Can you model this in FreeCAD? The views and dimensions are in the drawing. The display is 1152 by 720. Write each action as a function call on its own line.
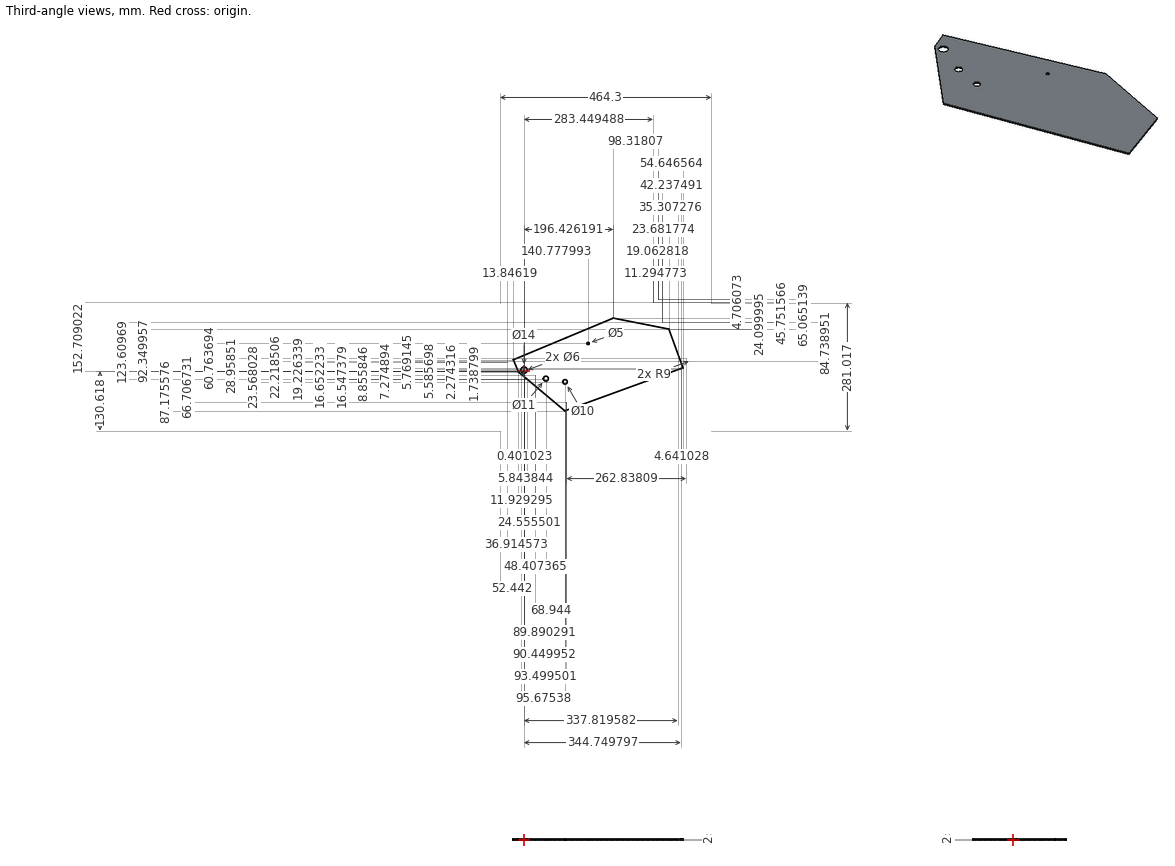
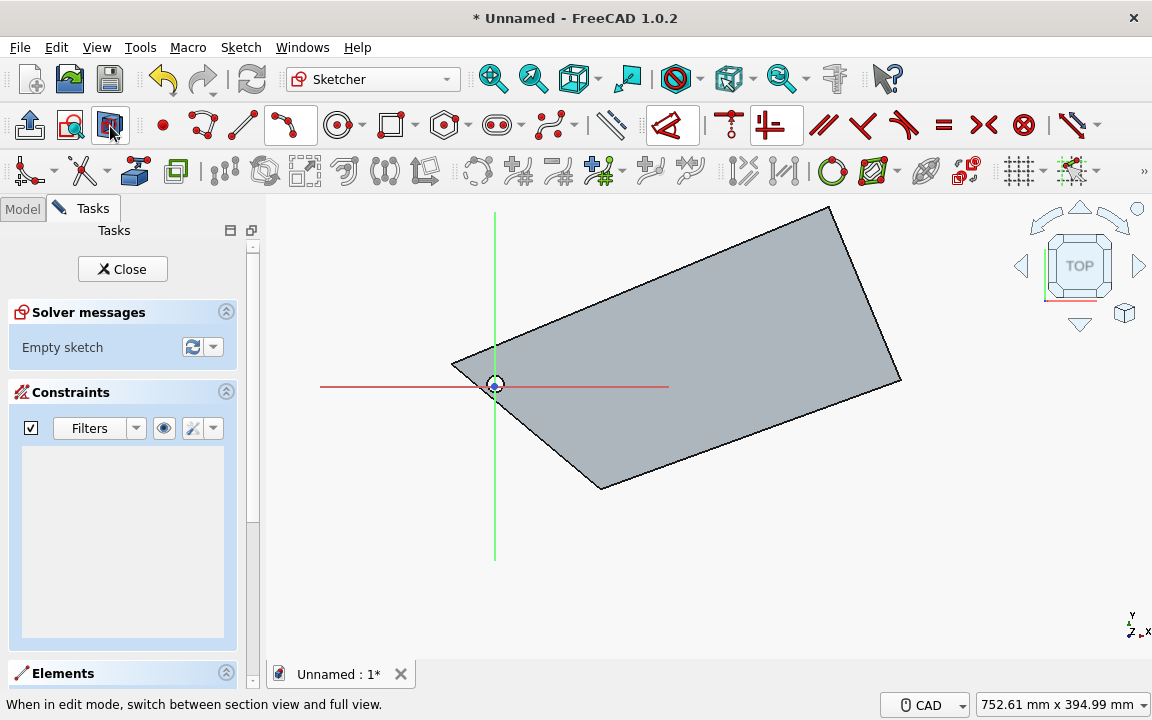
scroll(369, 631, down, 1)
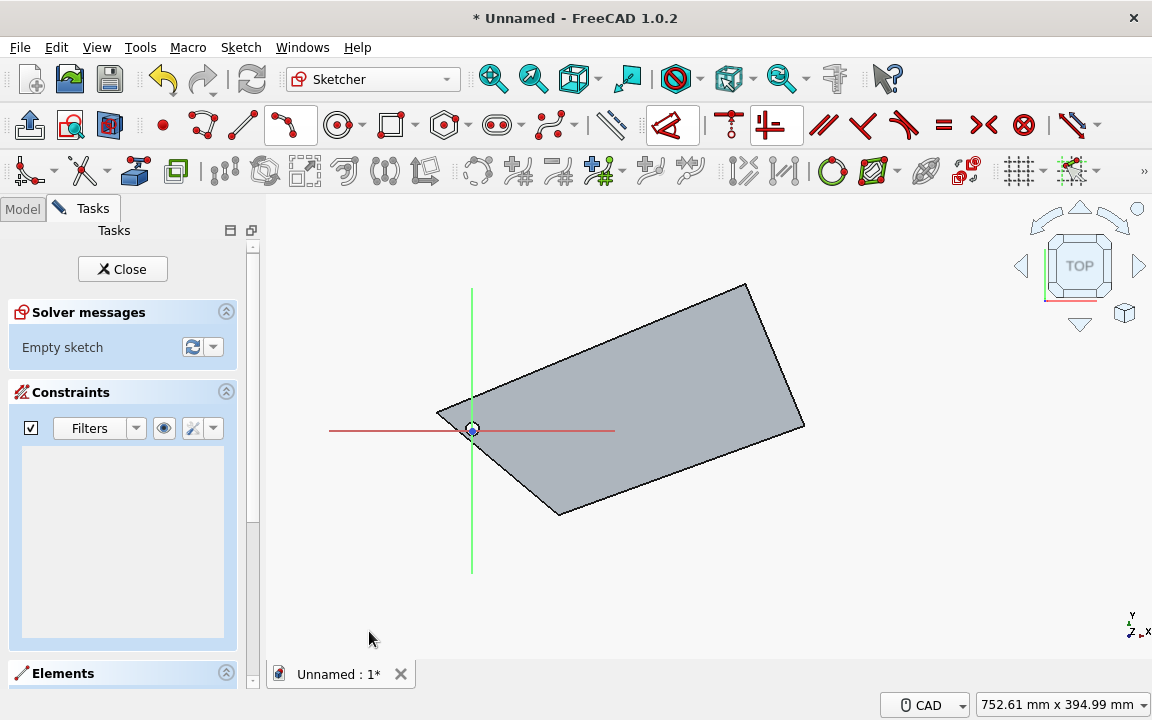
scroll(641, 222, up, 2)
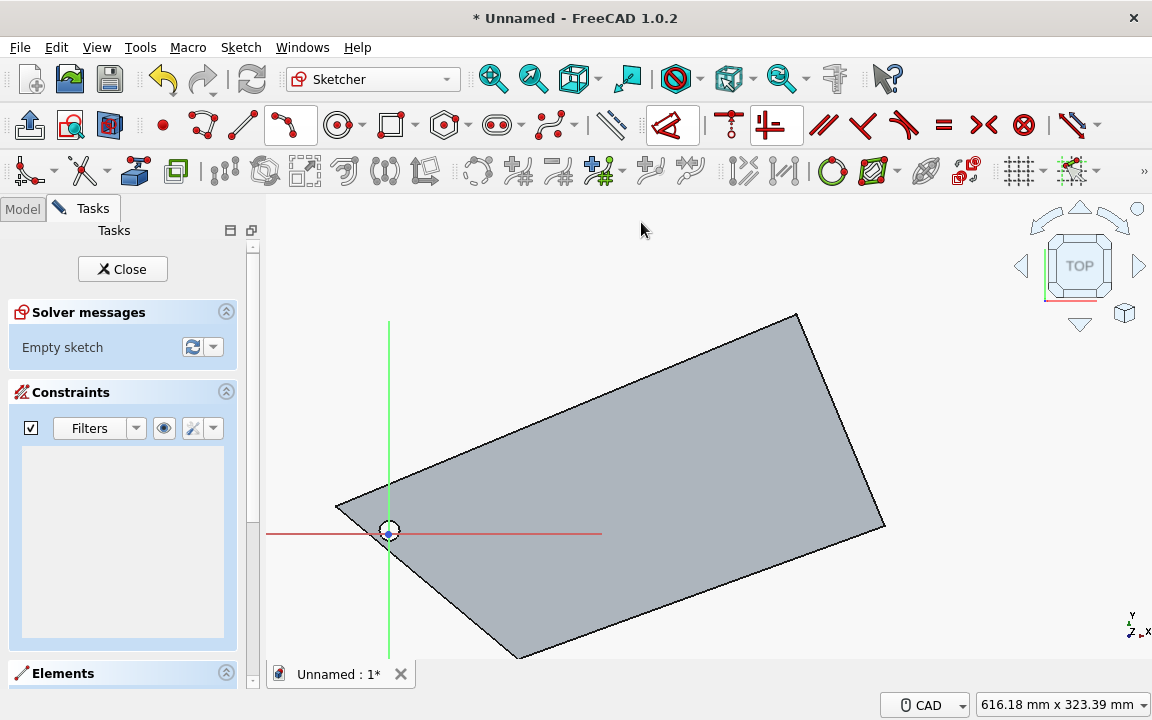
key(g)
key(m)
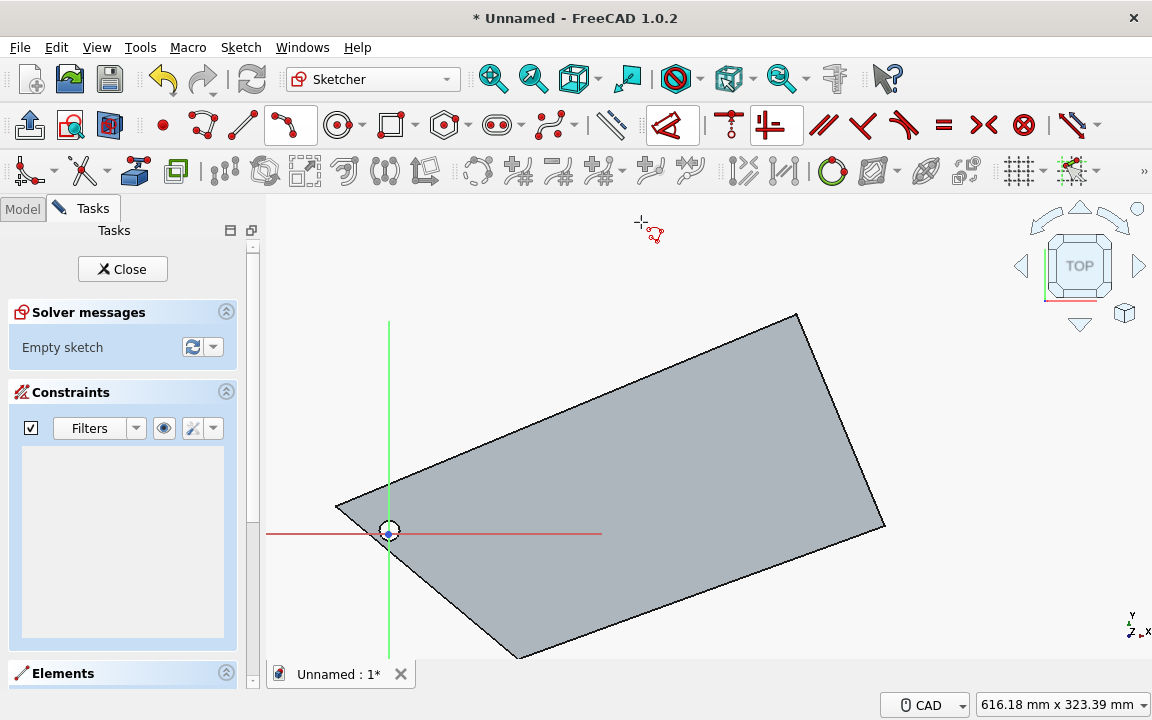
click(796, 314)
click(813, 308)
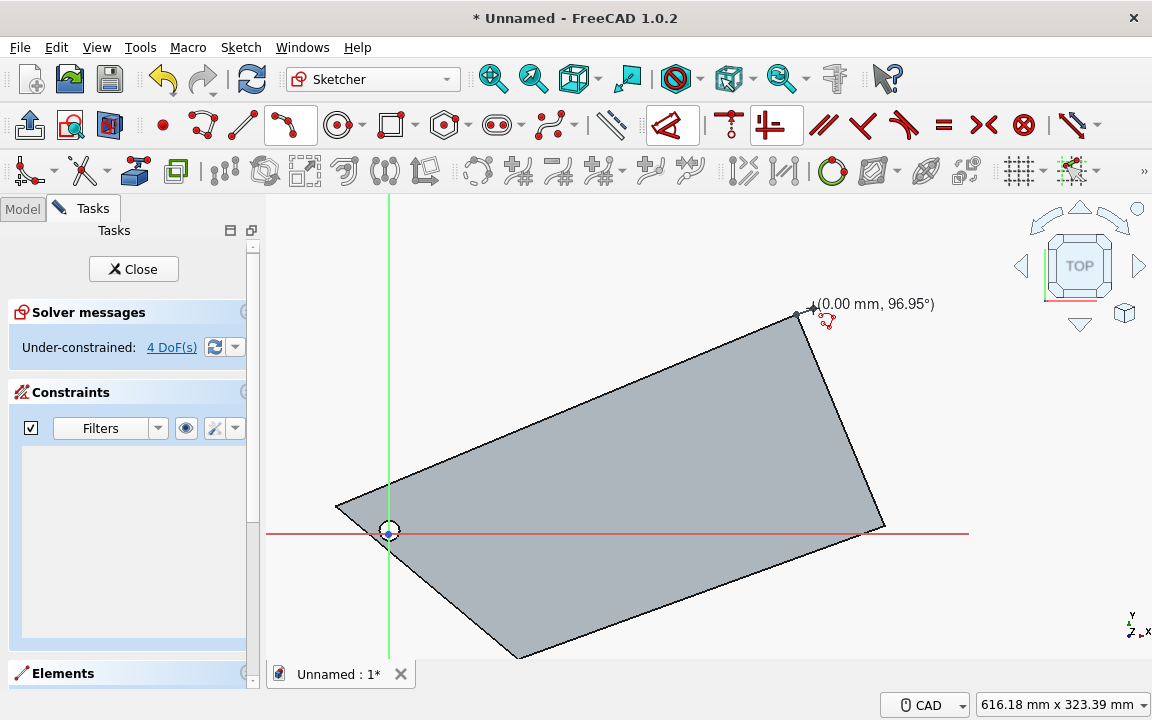
scroll(891, 524, up, 3)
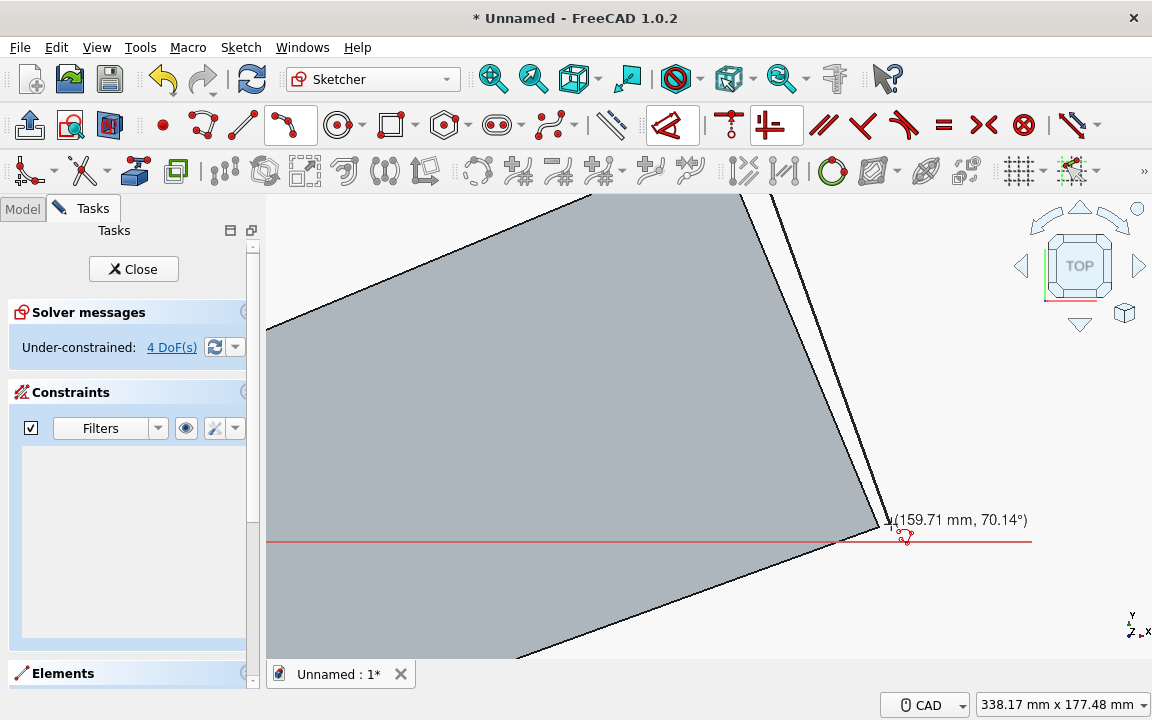
click(891, 523)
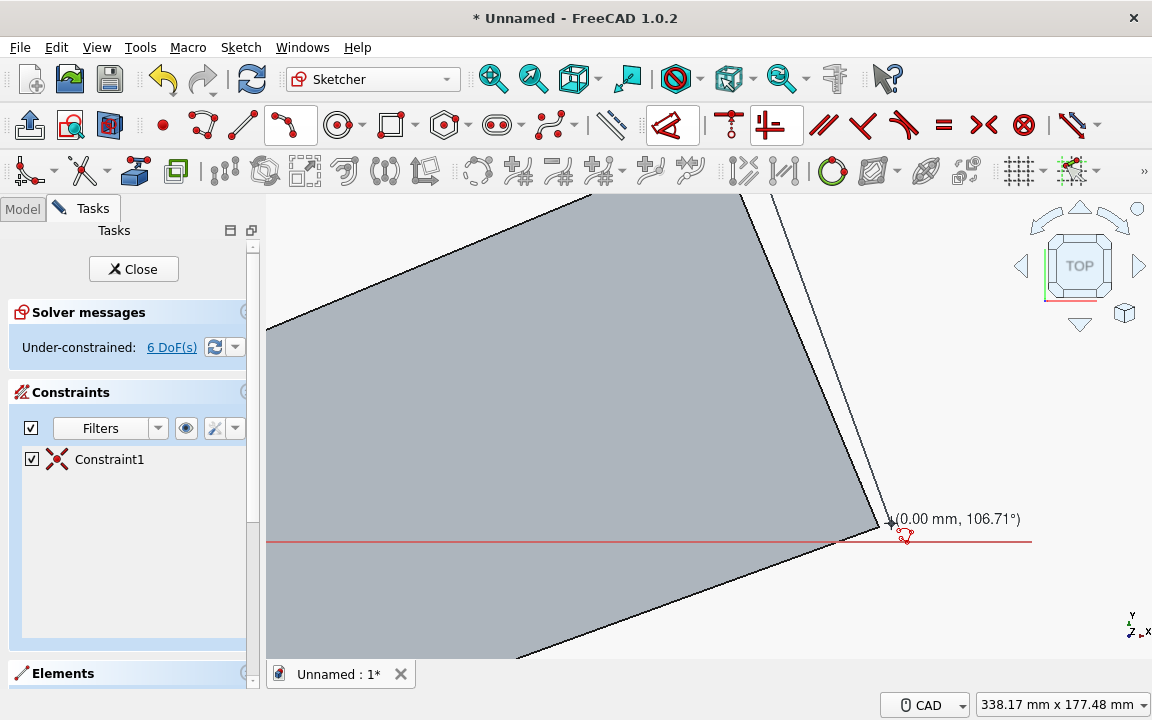
scroll(879, 527, up, 2)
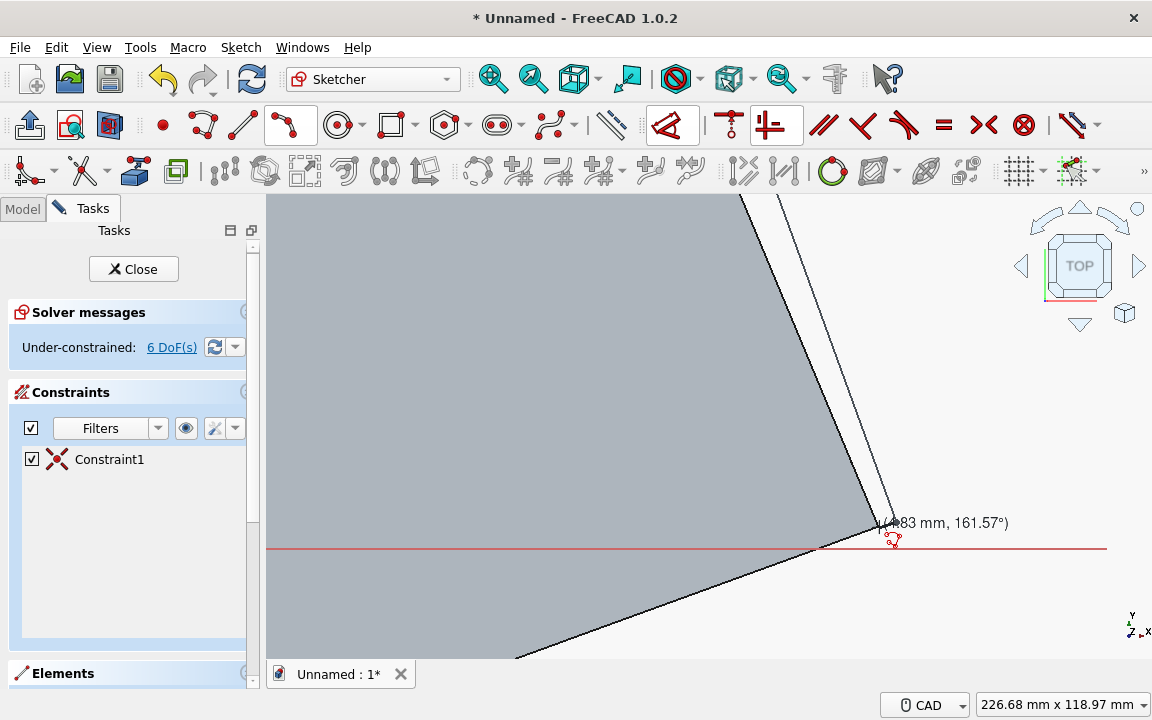
click(878, 527)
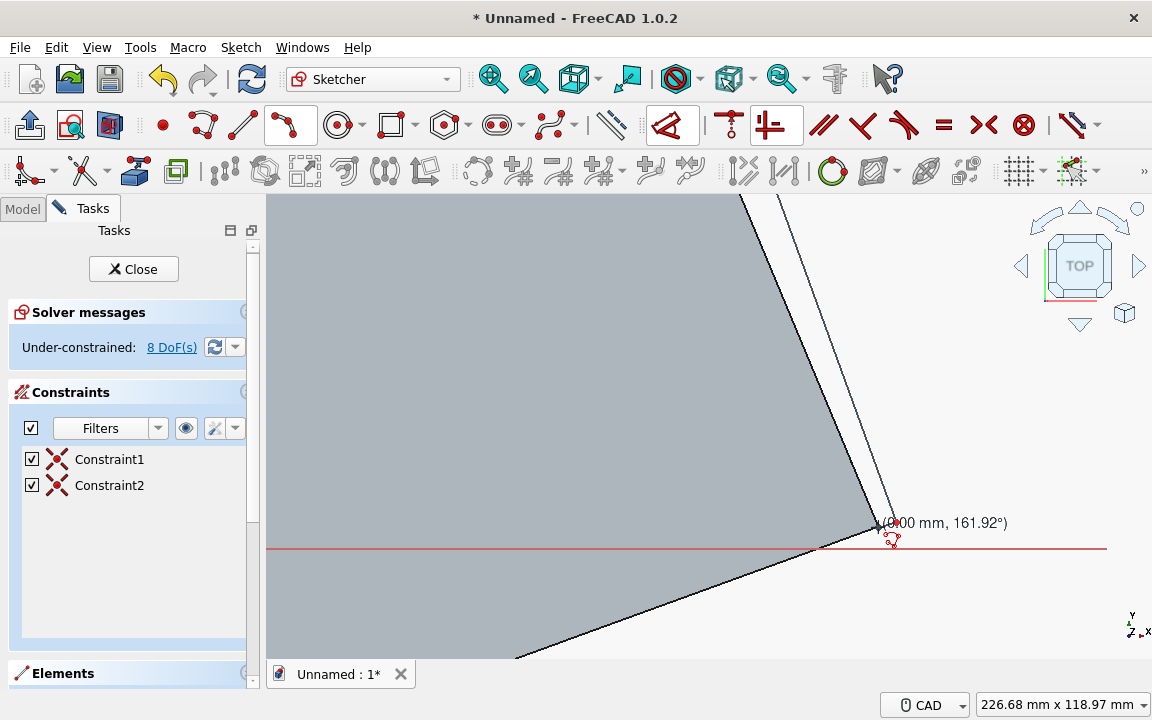
scroll(889, 535, down, 5)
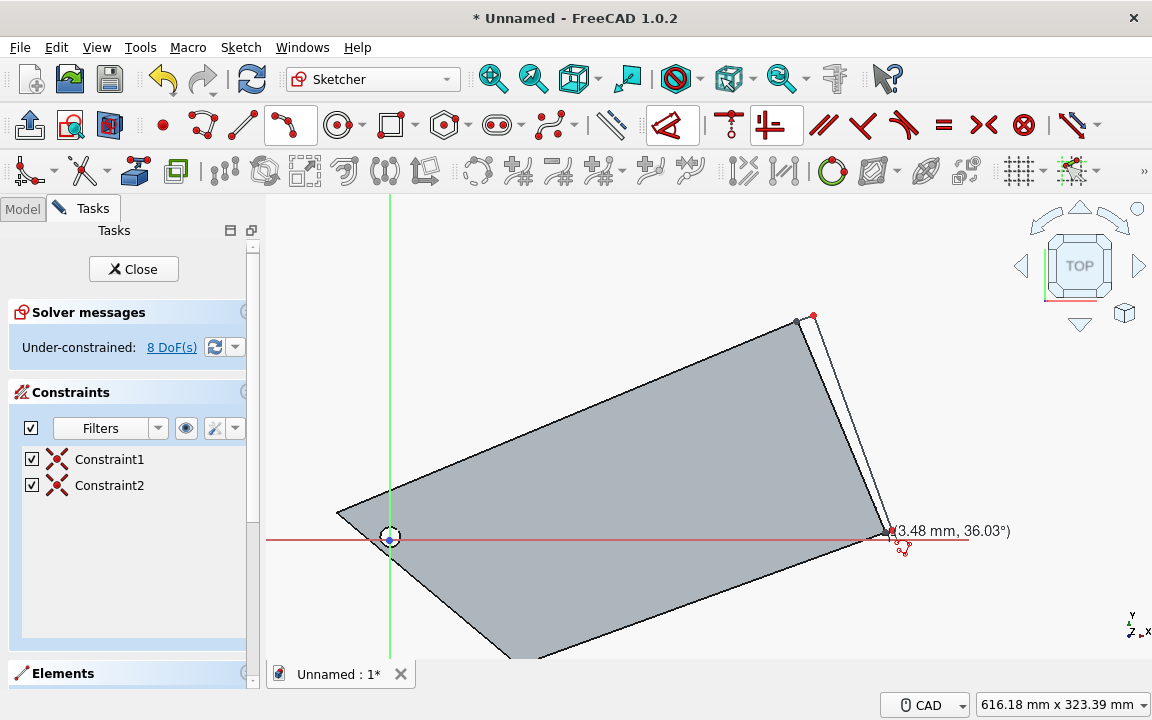
scroll(797, 321, up, 3)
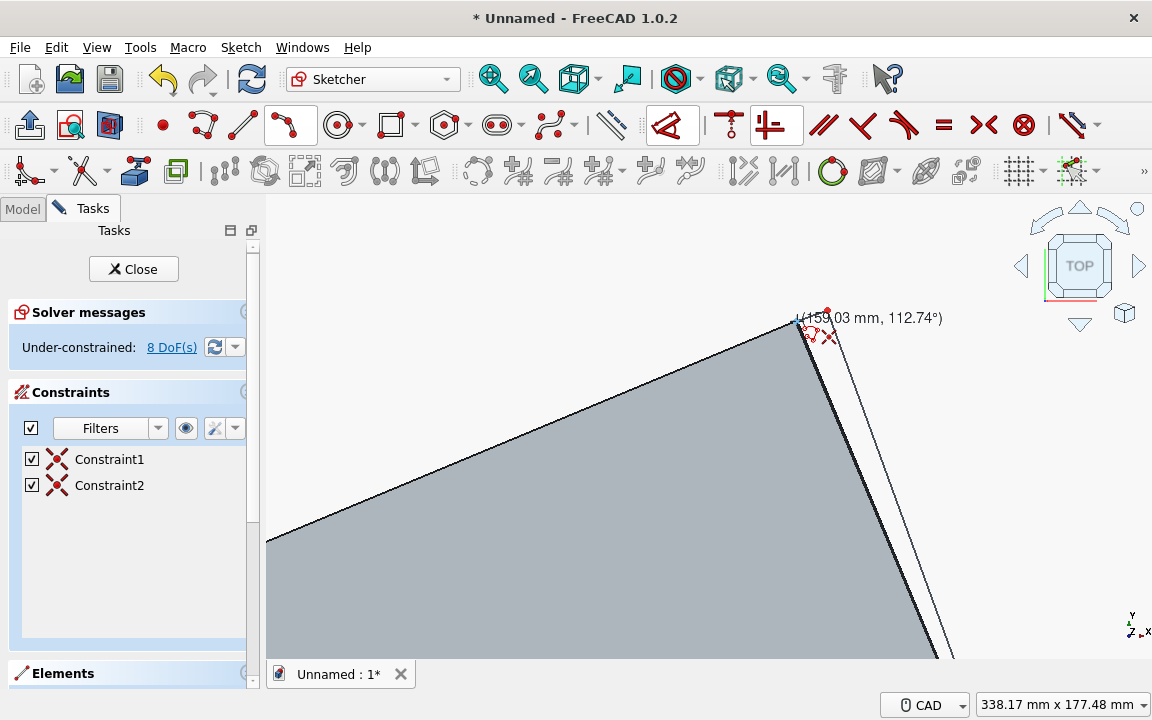
click(796, 322)
key(Escape)
key(Escape)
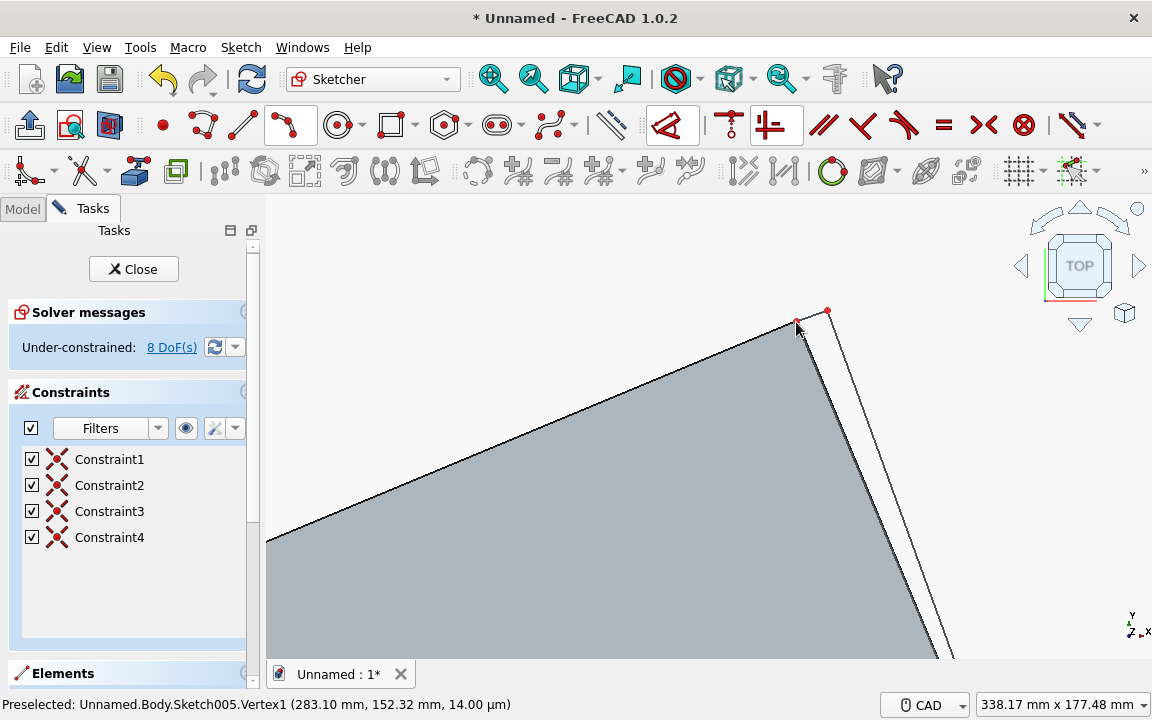
scroll(796, 320, down, 3)